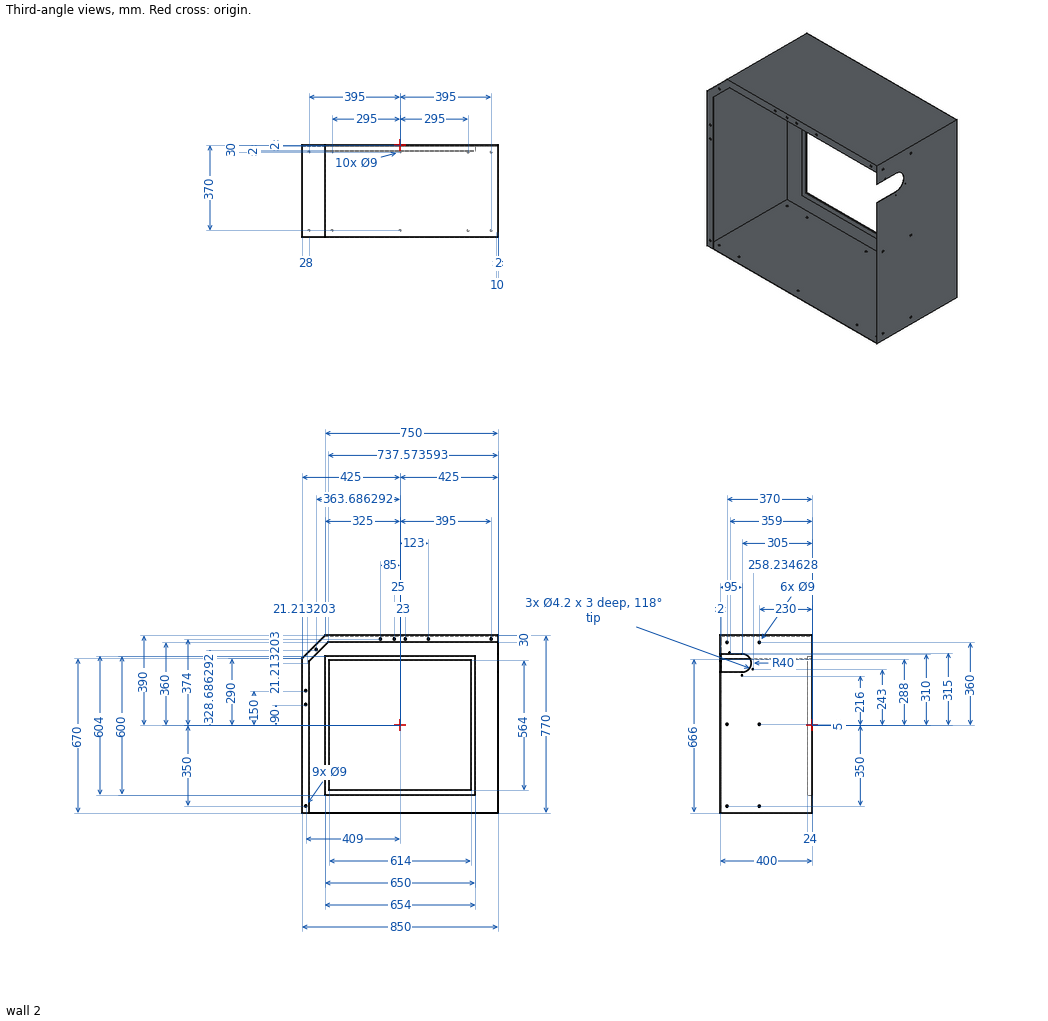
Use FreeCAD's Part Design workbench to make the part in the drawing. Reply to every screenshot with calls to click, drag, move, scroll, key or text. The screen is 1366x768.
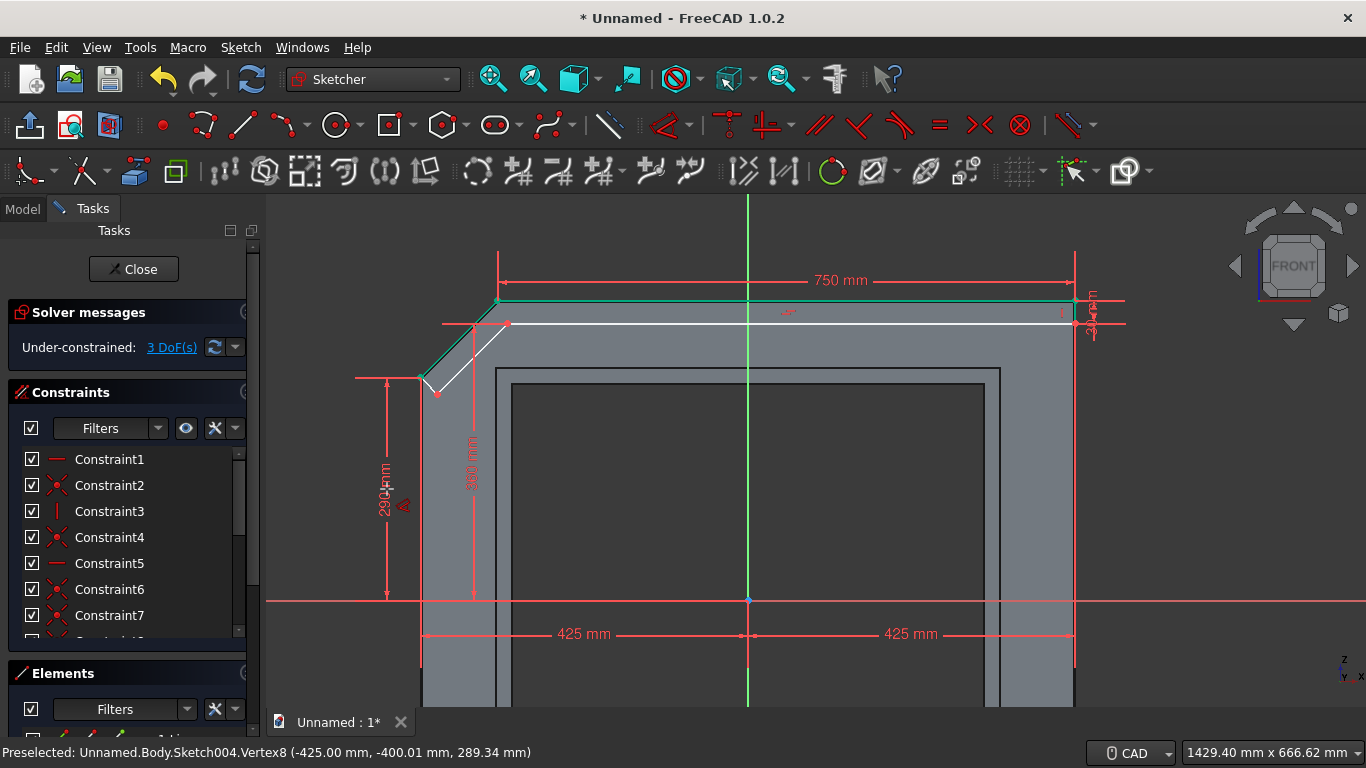
click(678, 324)
click(791, 358)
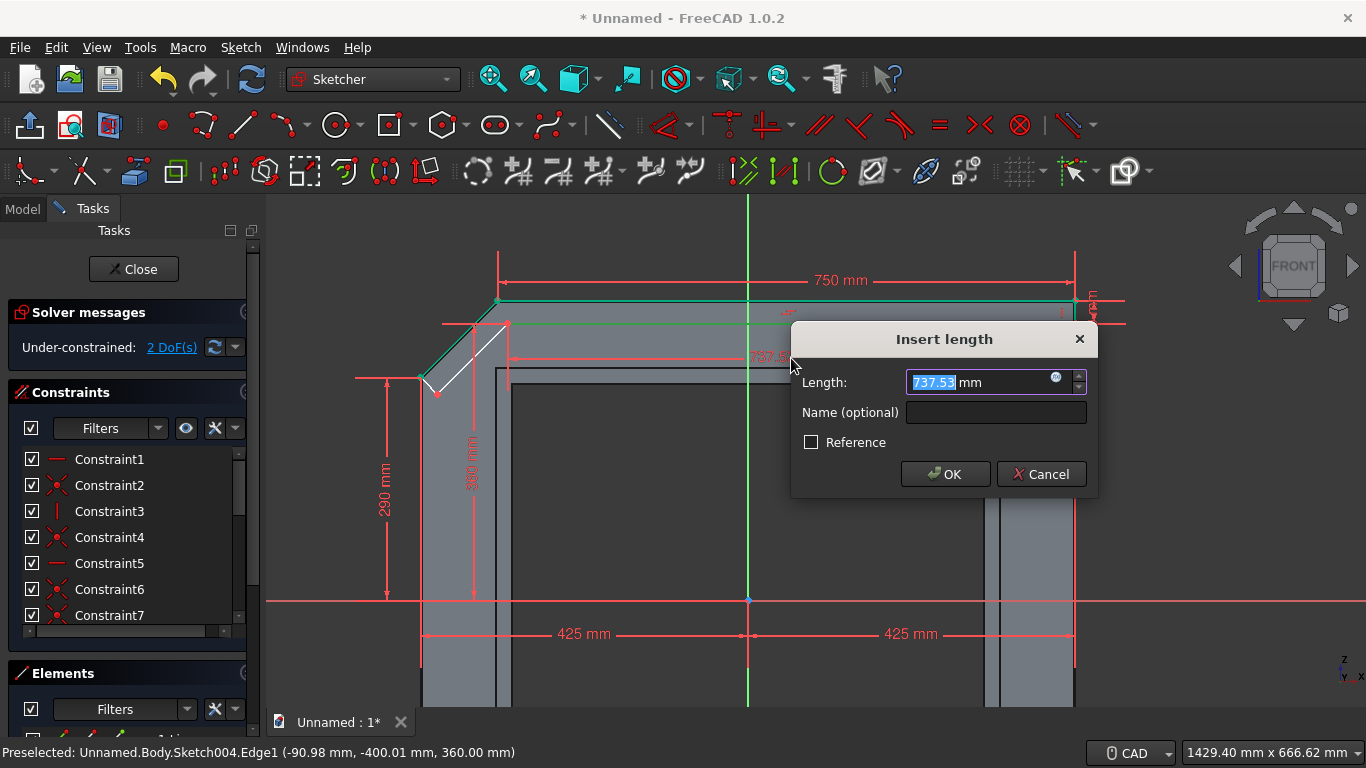
text(737.573593)
key(Return)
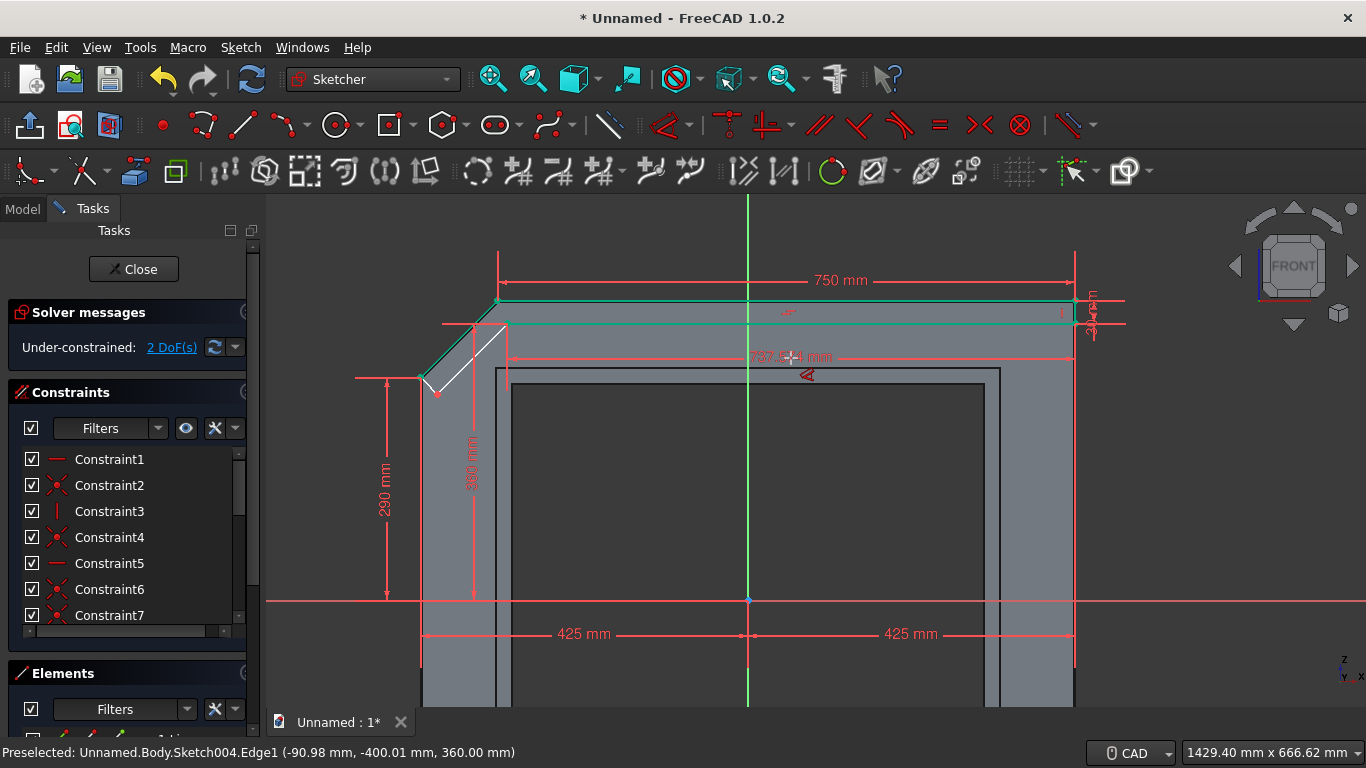
scroll(427, 384, up, 5)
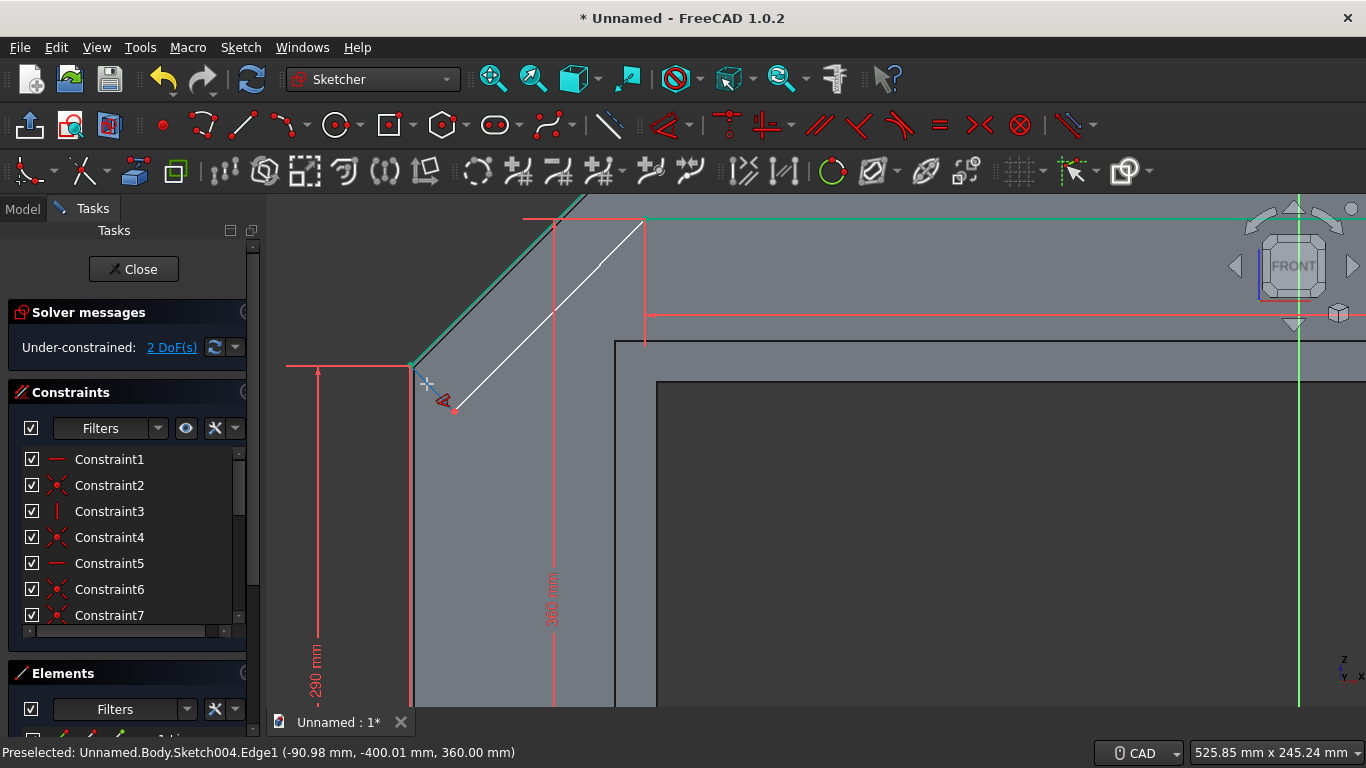
click(428, 384)
click(422, 332)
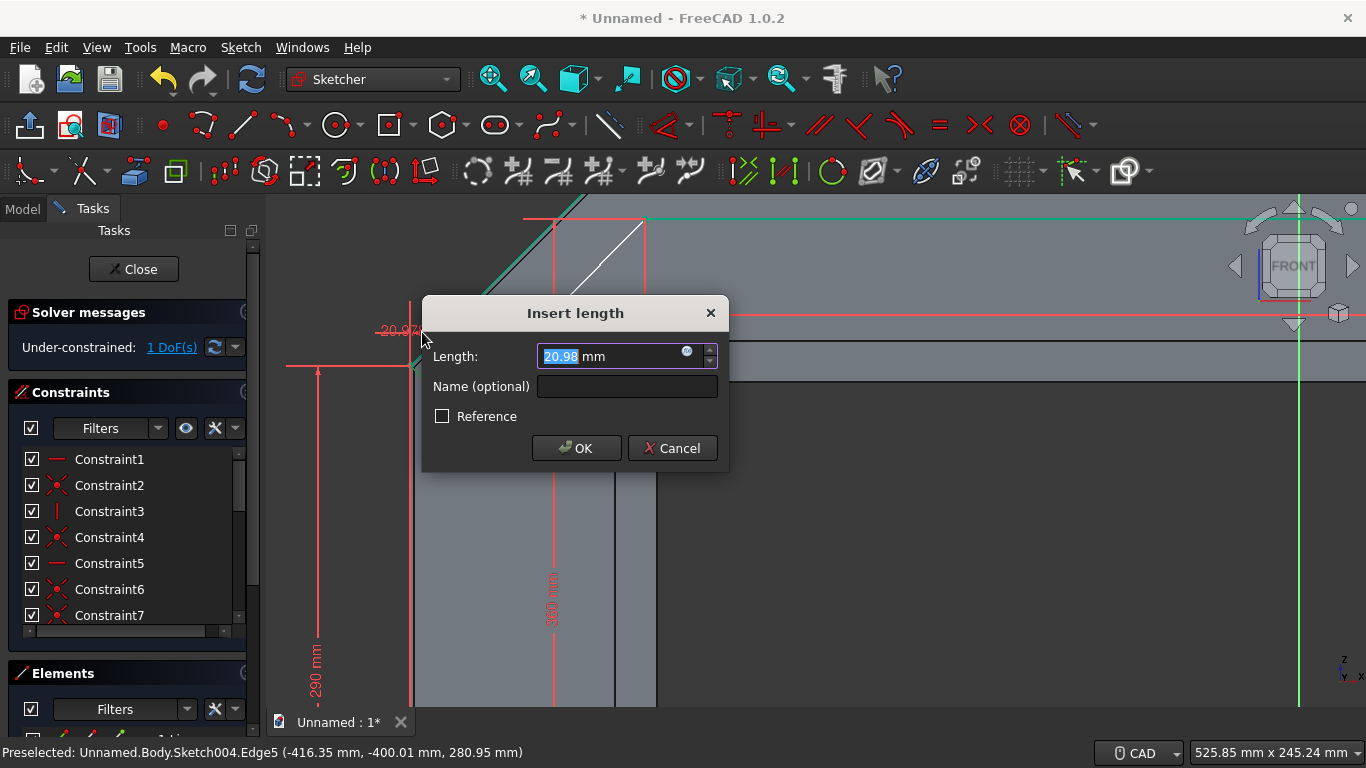
text(21.213203)
key(Return)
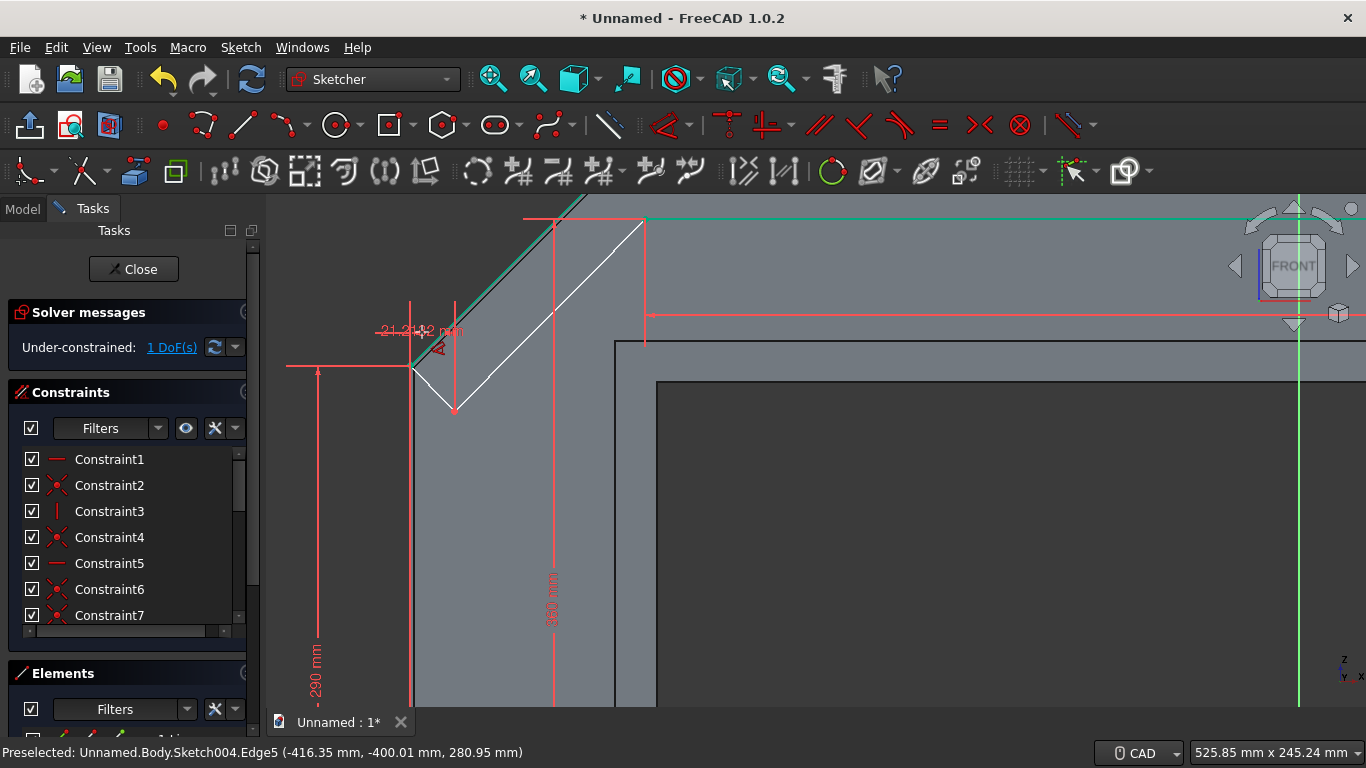
click(424, 379)
click(376, 389)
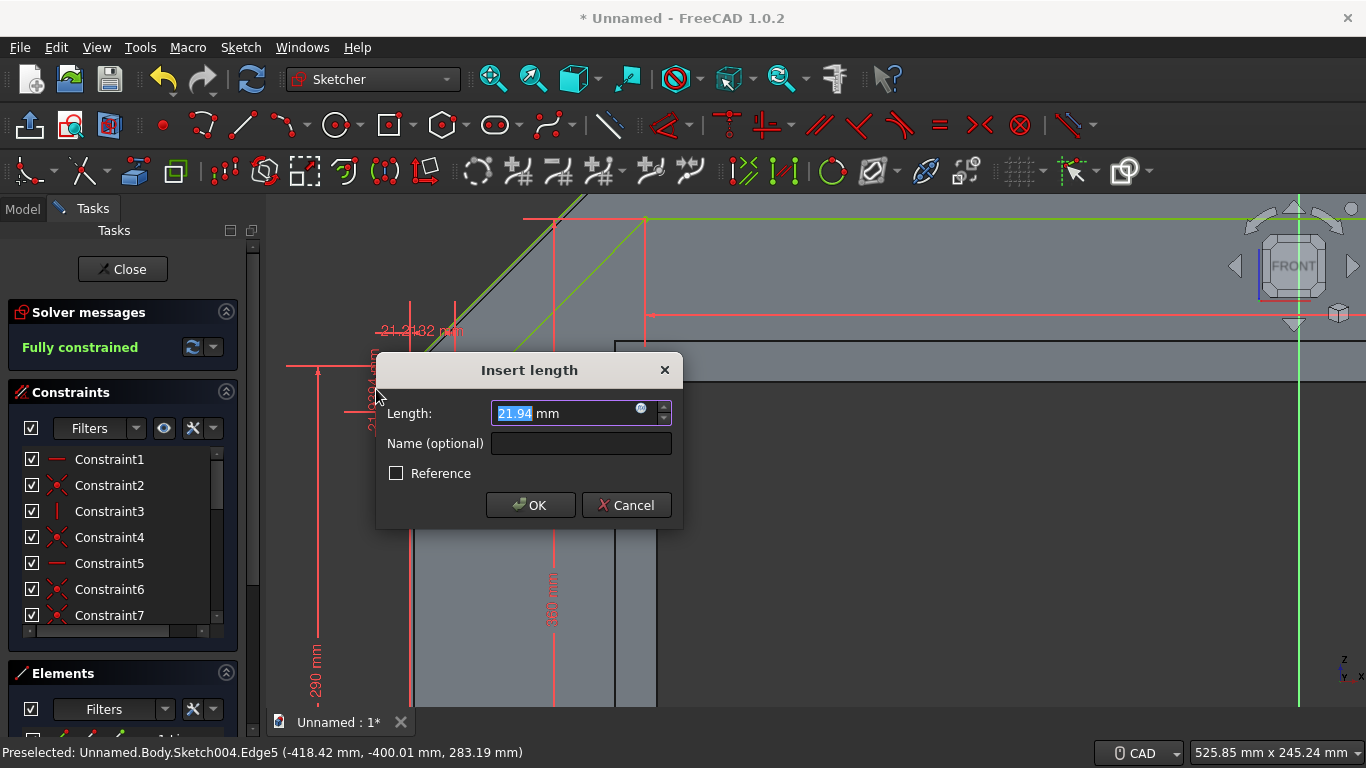
text(21.213203)
key(Return)
key(Escape)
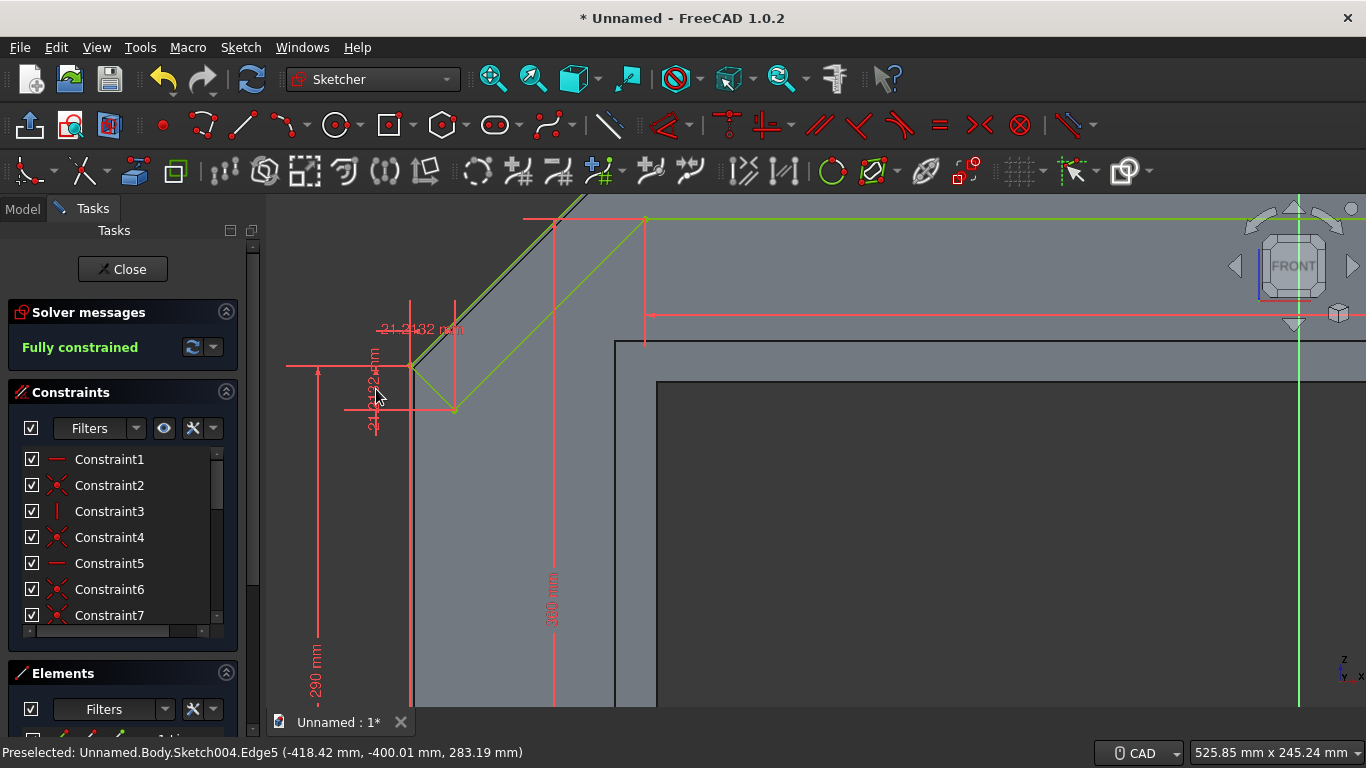
click(123, 269)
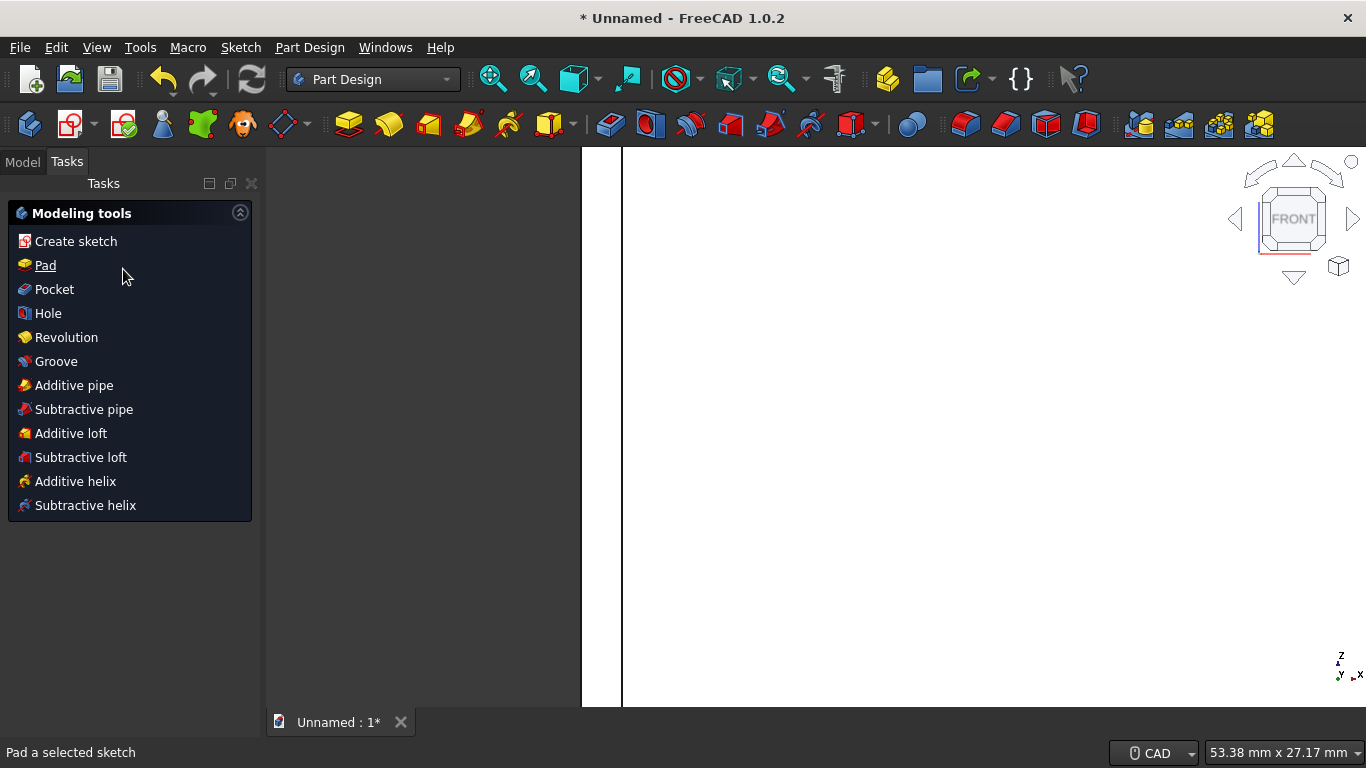
click(350, 124)